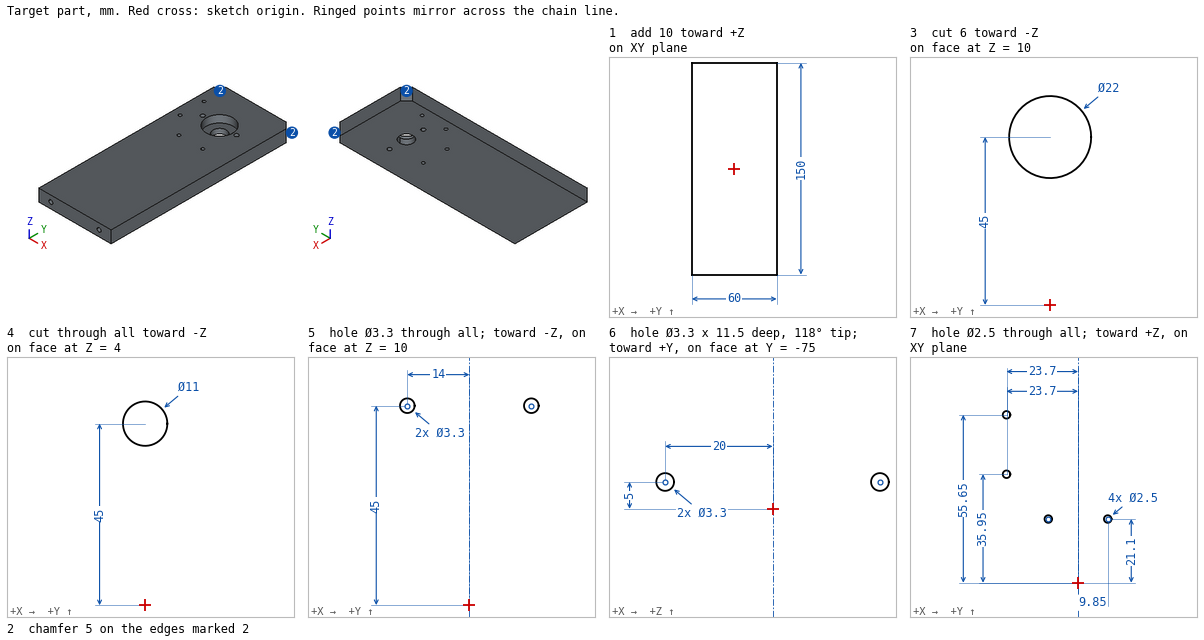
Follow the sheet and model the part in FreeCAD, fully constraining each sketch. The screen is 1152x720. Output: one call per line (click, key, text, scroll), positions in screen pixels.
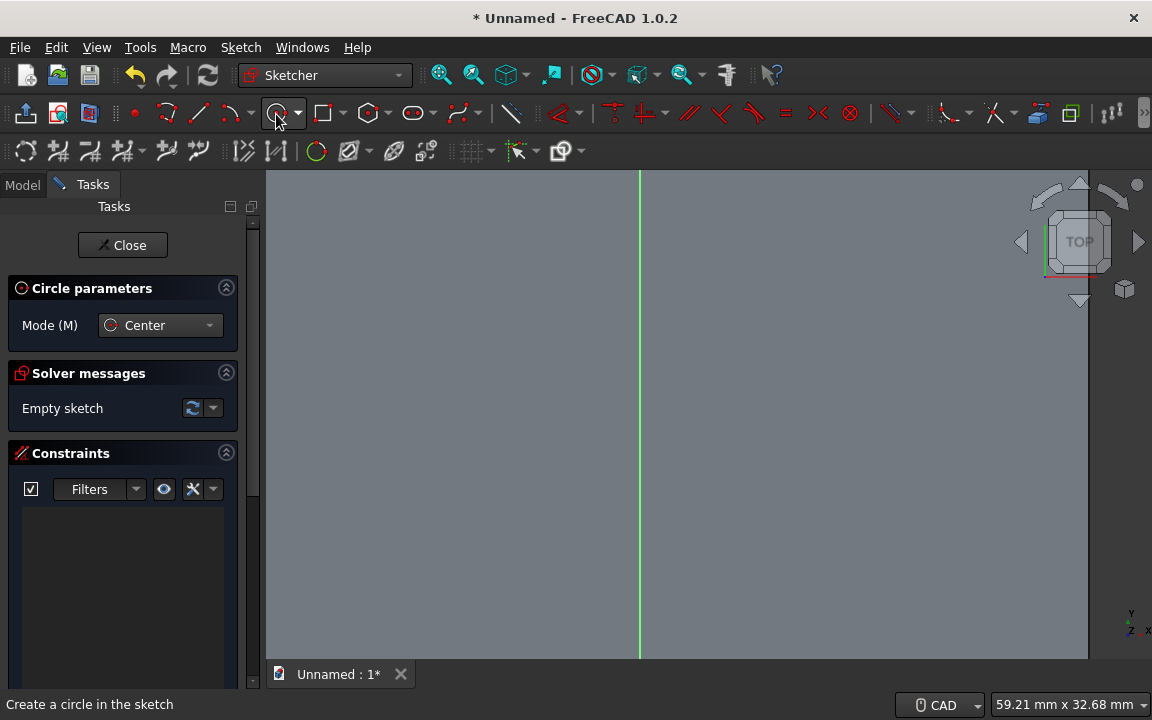
click(640, 415)
click(756, 298)
key(Escape)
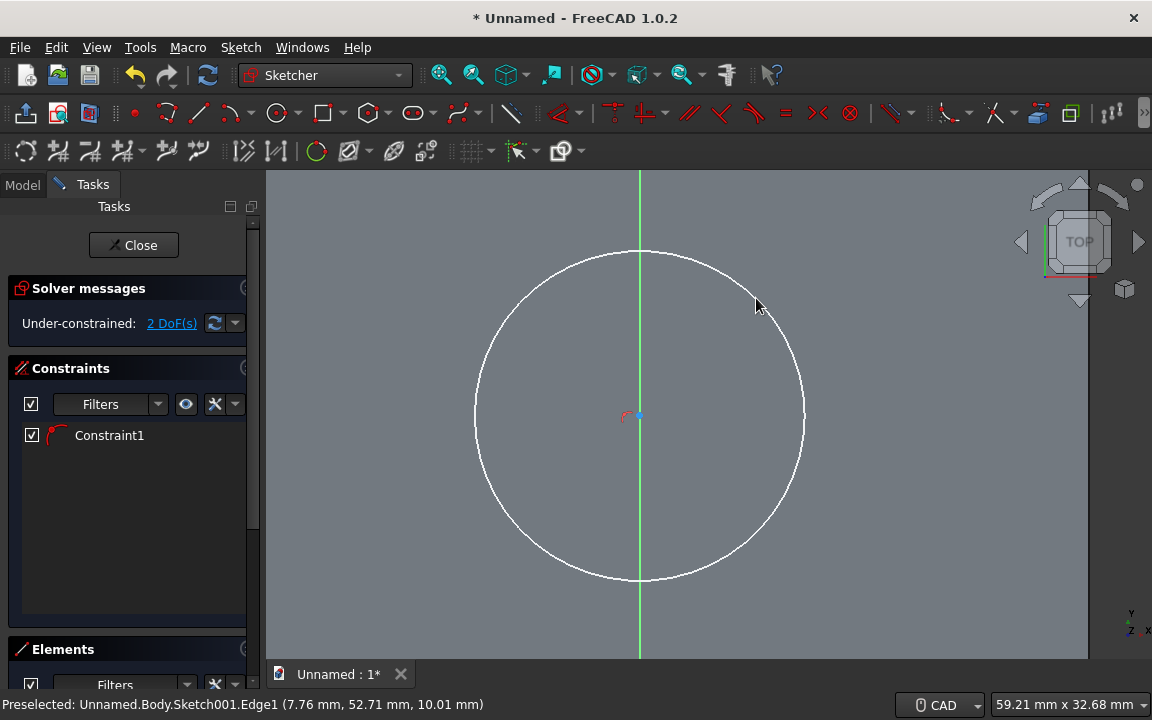
click(558, 114)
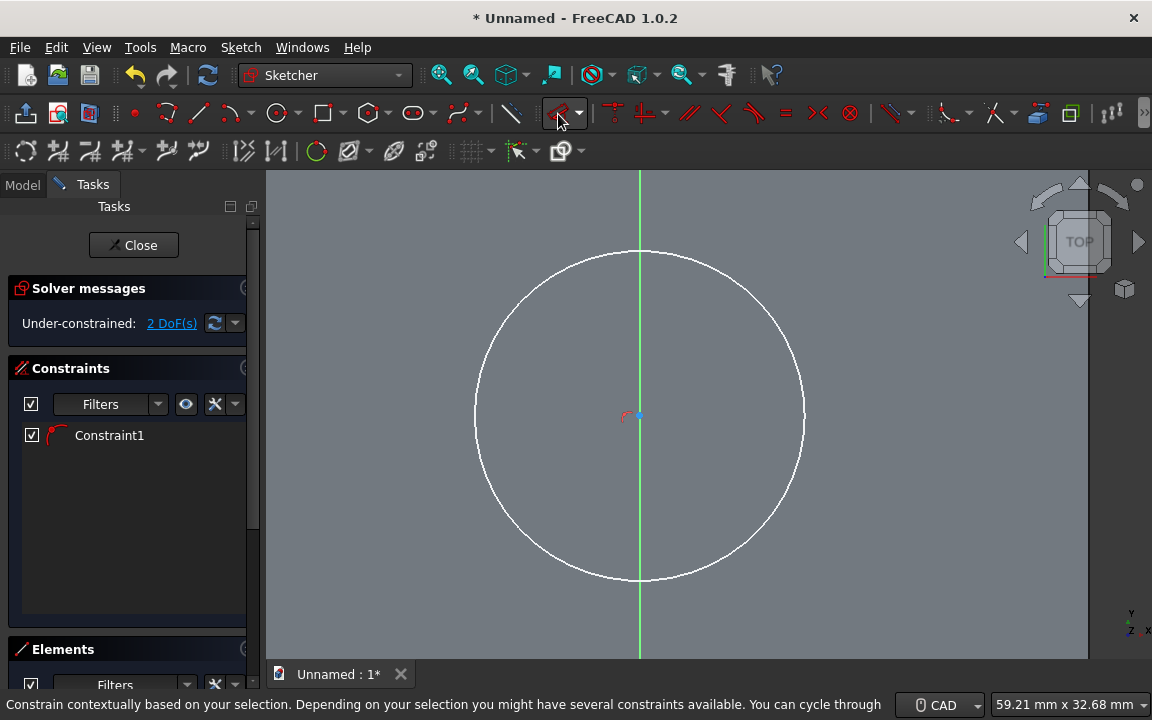
click(756, 299)
click(779, 276)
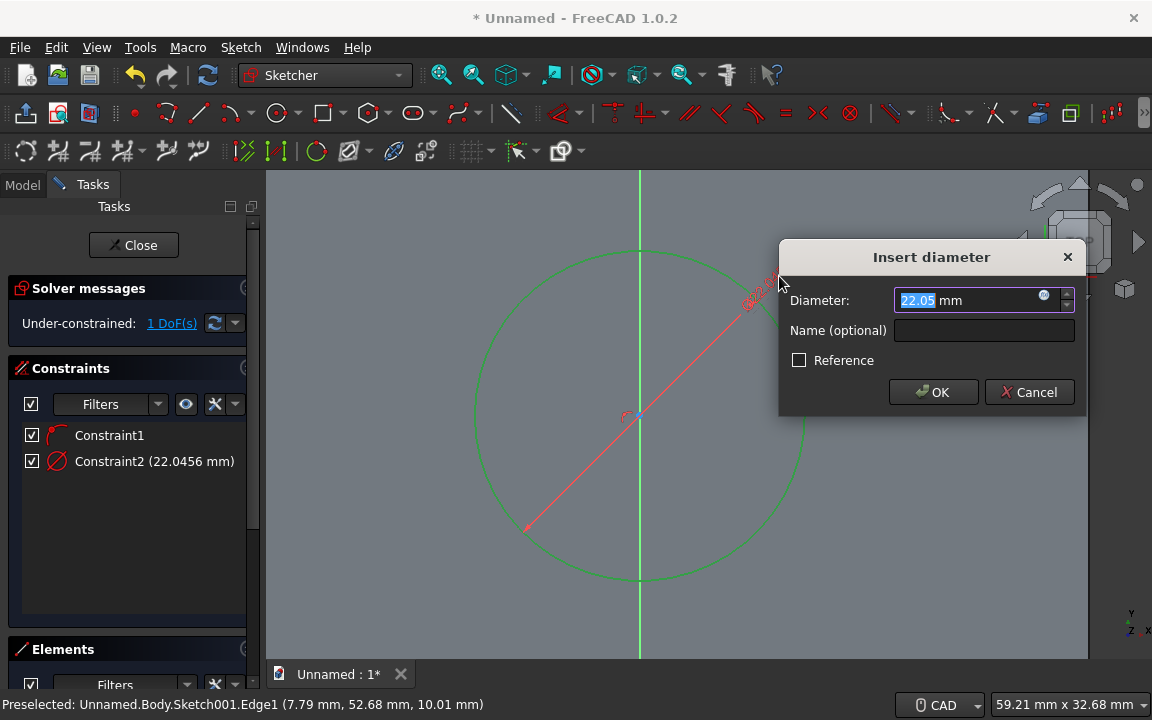
text(22)
key(Return)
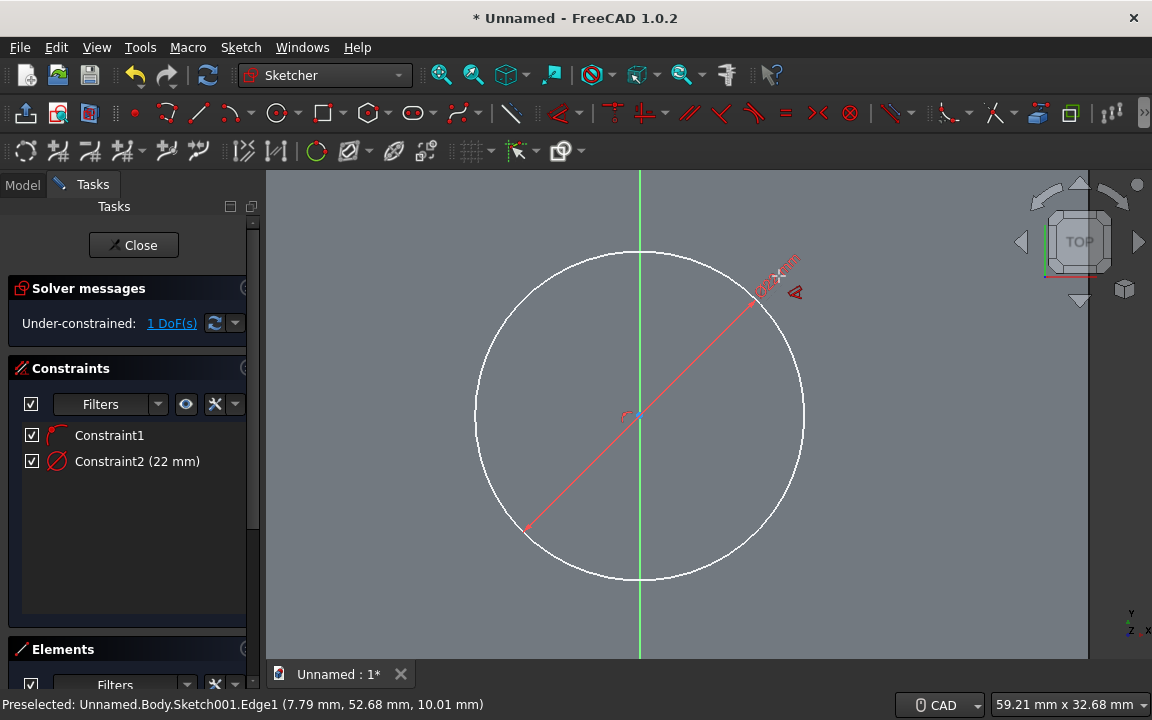
click(640, 416)
click(674, 524)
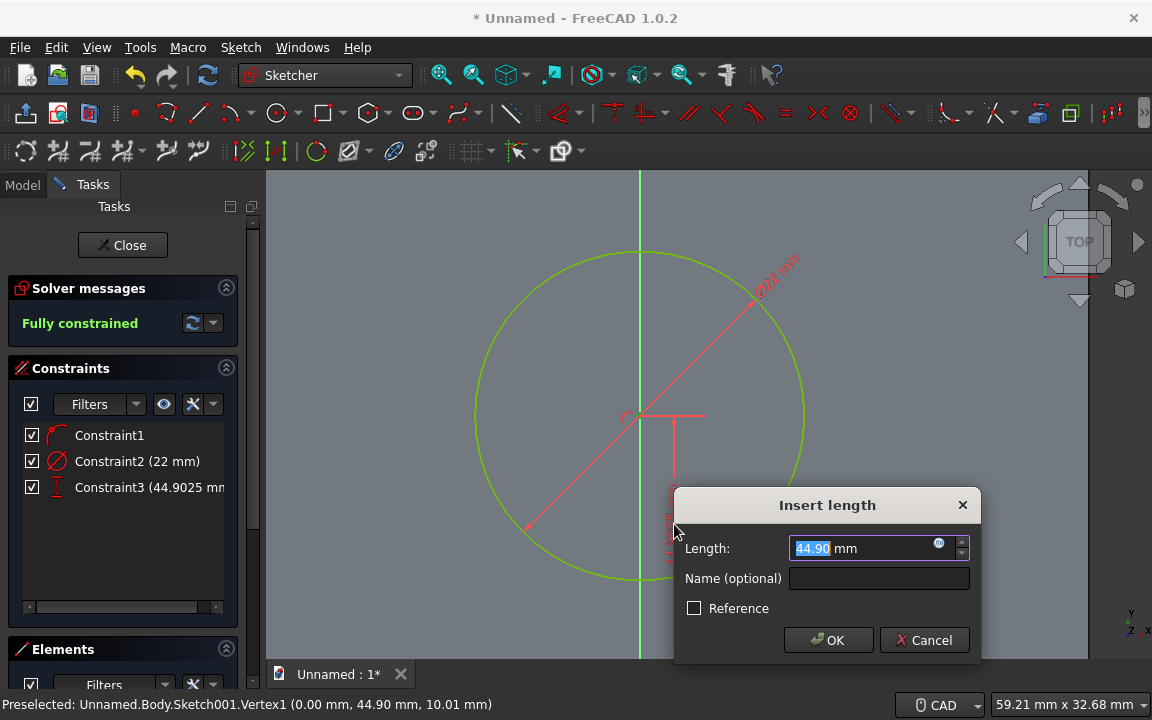
text(45)
key(Return)
key(Escape)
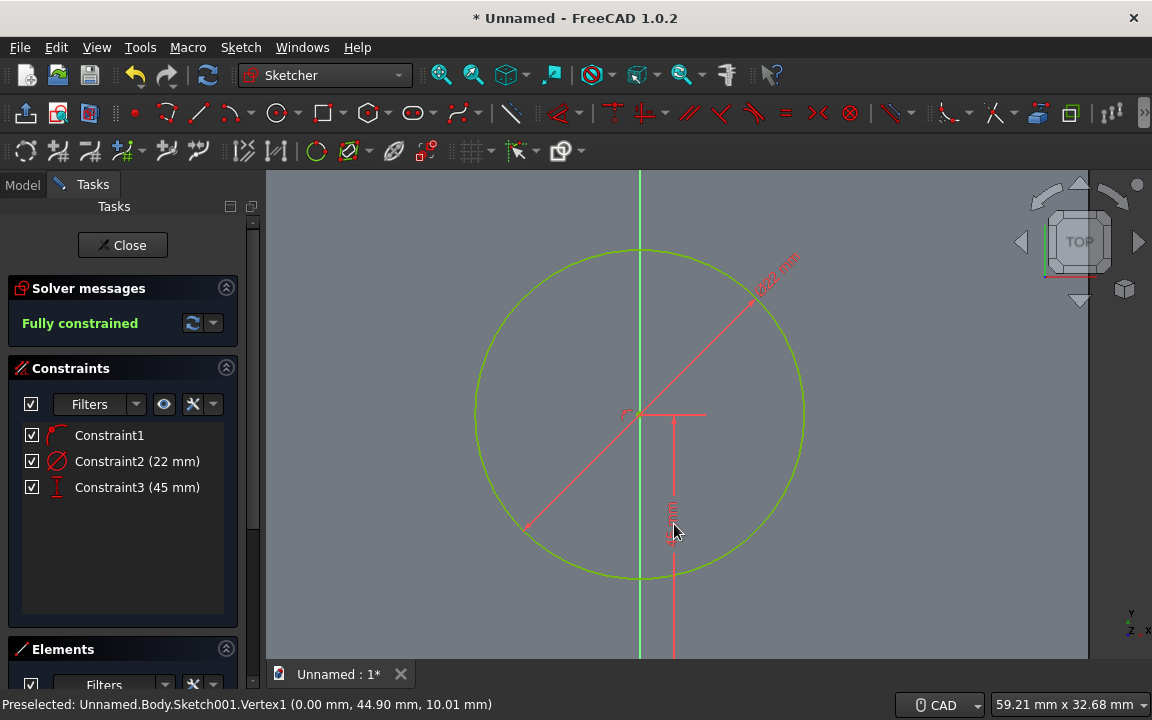
click(123, 245)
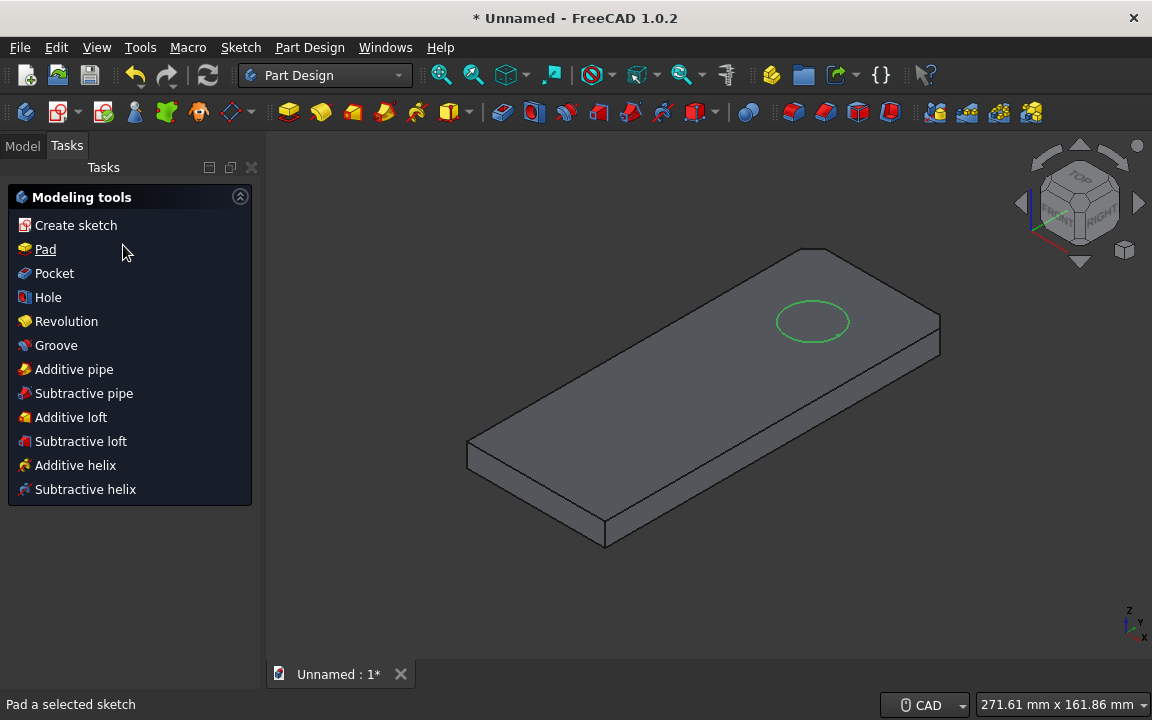
click(504, 112)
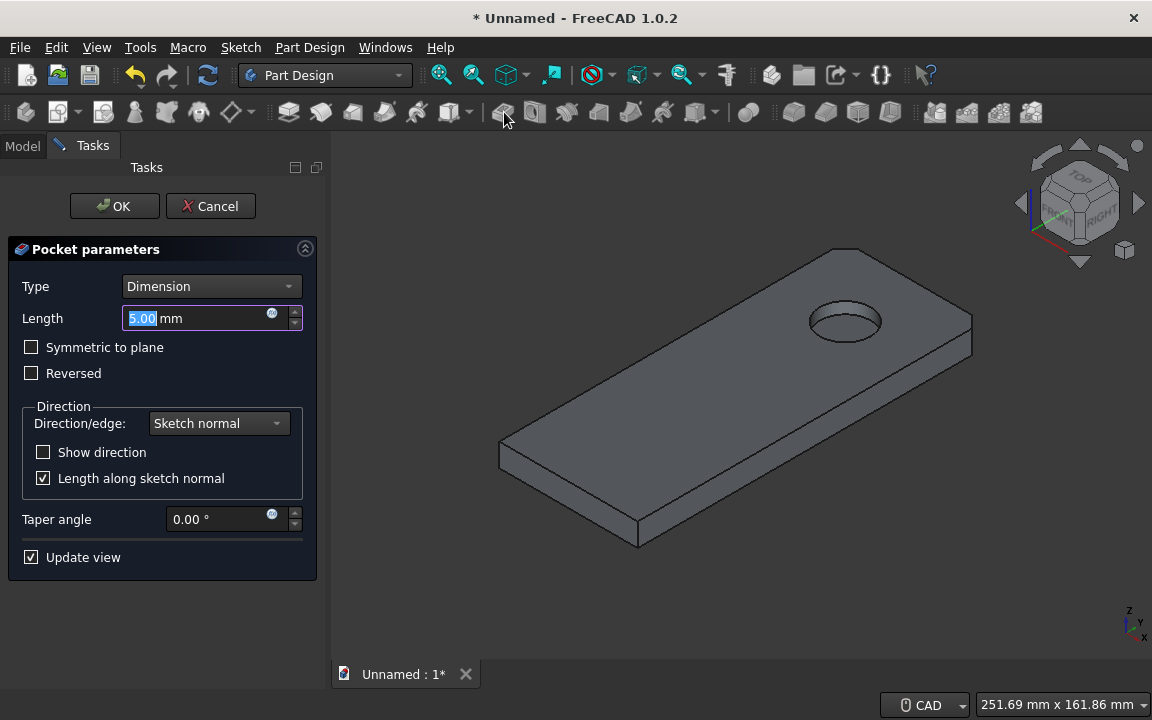
text(6)
key(Tab)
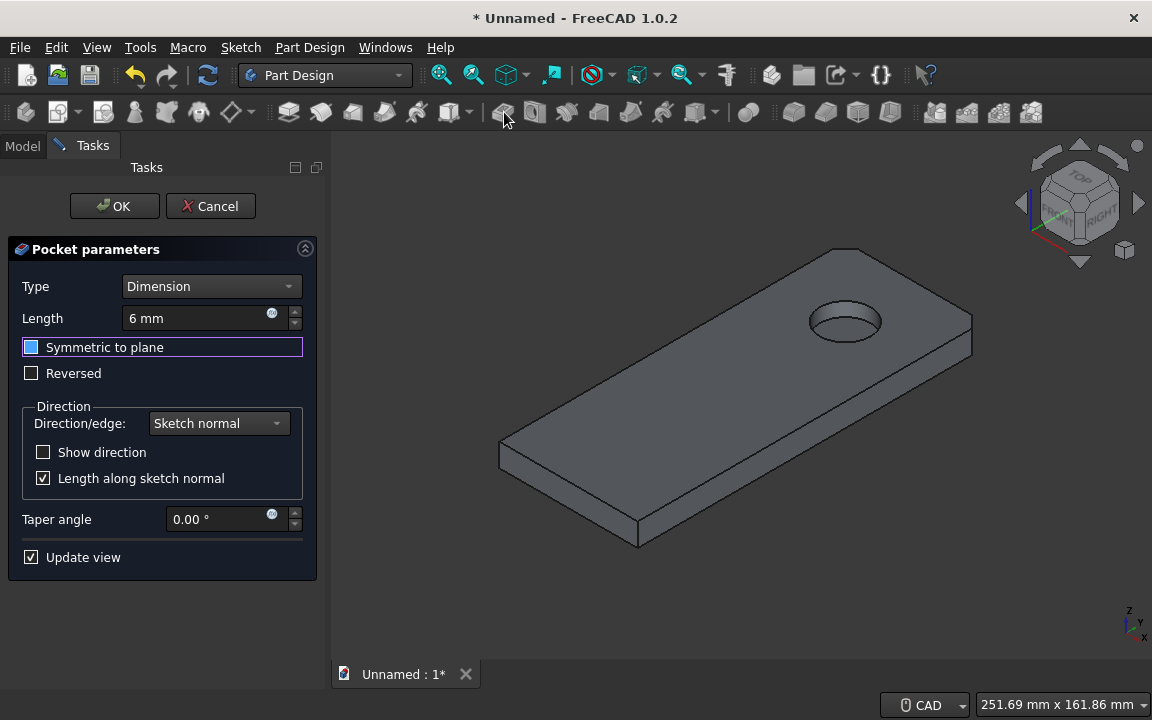
click(115, 206)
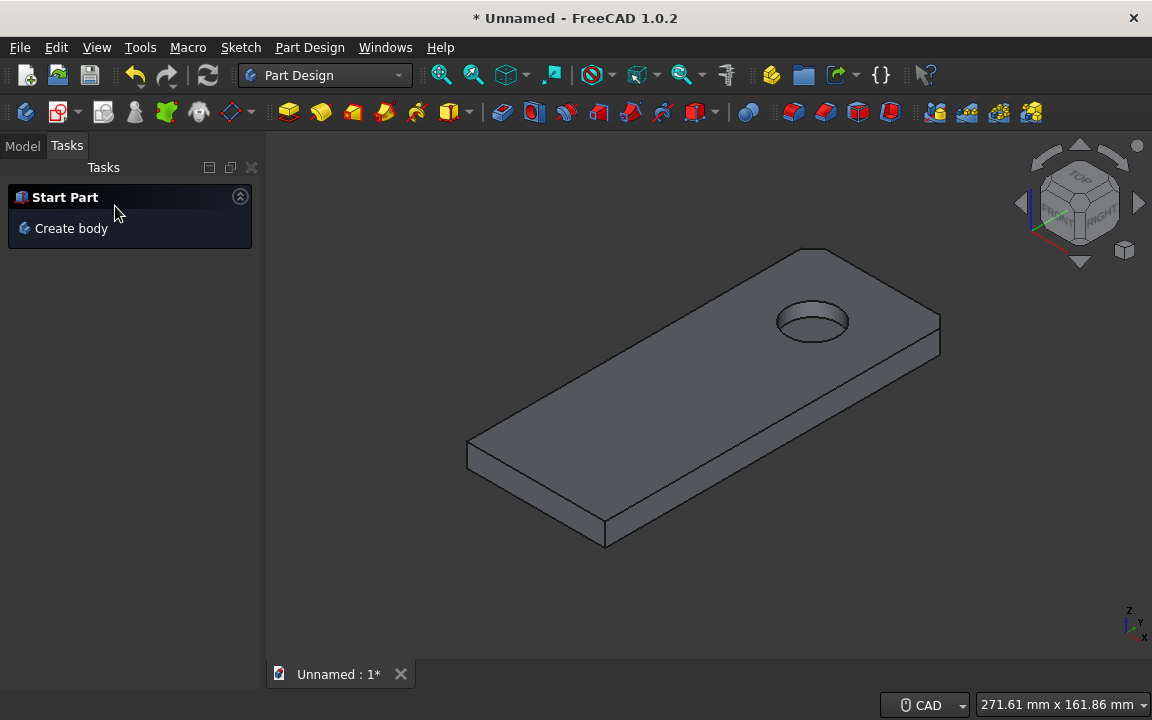
click(813, 328)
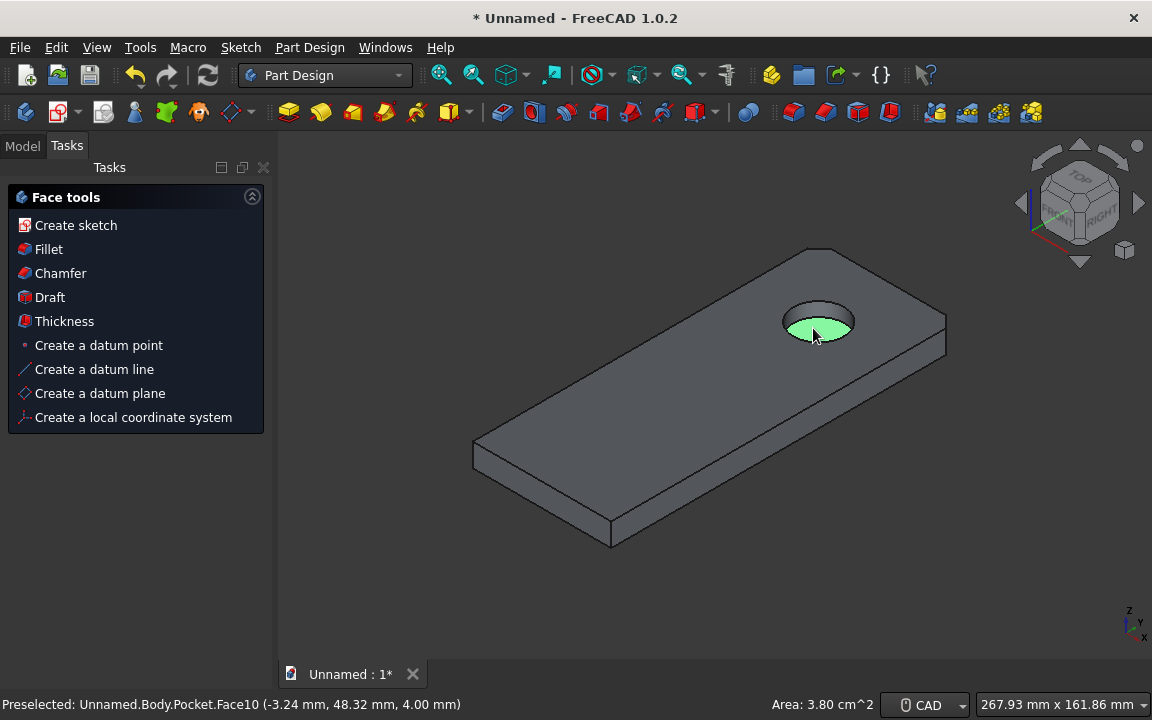
click(58, 112)